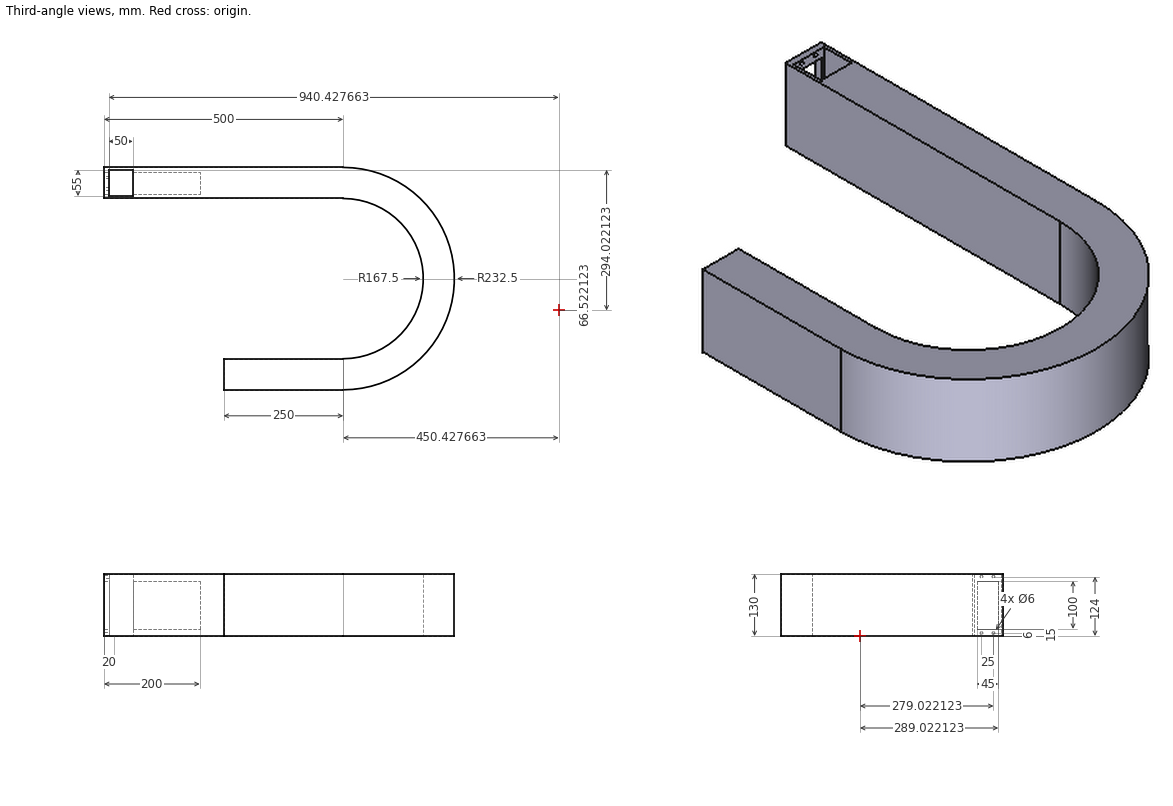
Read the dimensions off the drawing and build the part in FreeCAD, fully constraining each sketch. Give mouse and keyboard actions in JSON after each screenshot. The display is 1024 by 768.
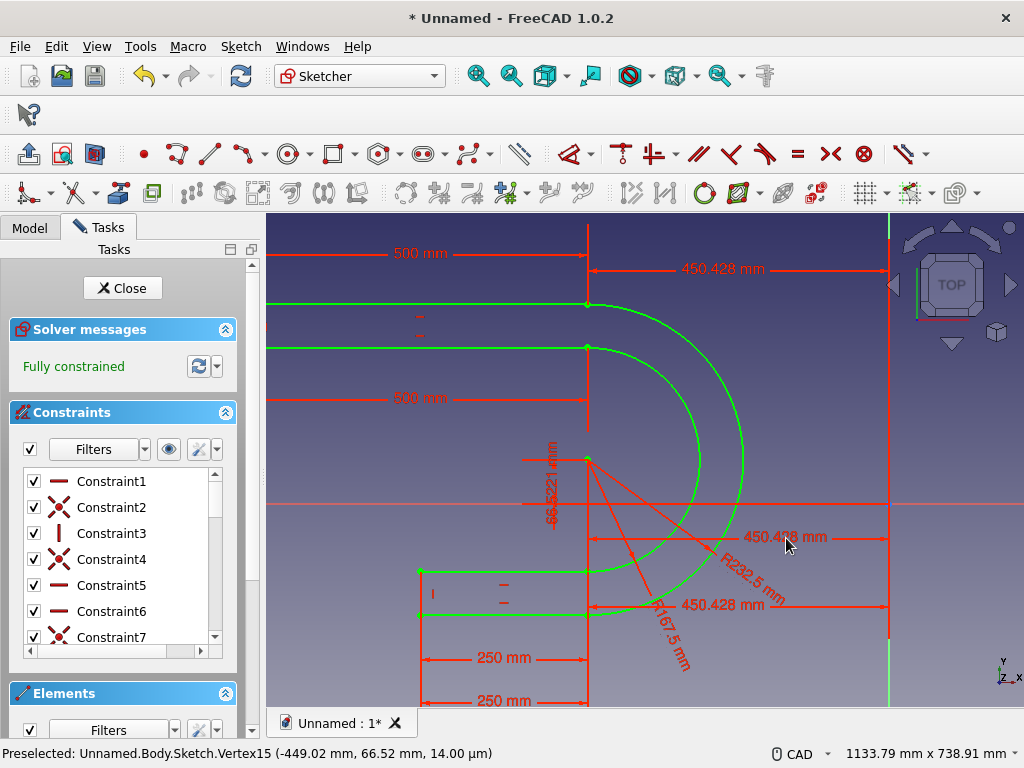
{"action": "left_click", "coordinate": [123, 288]}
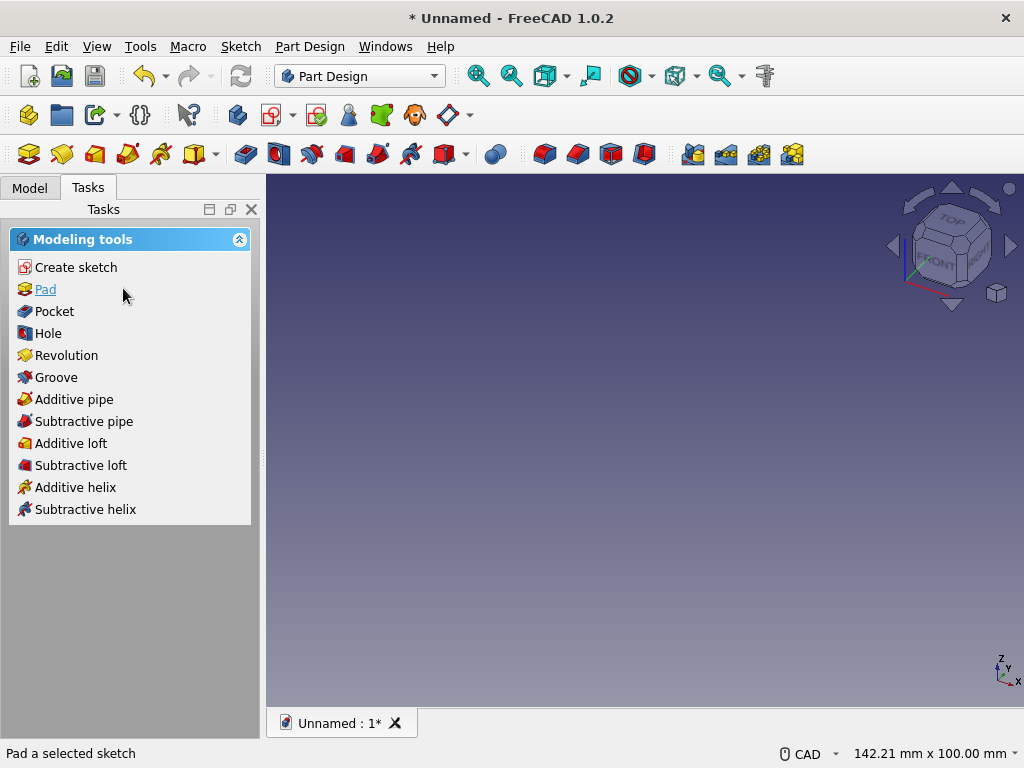
{"action": "left_click", "coordinate": [29, 154]}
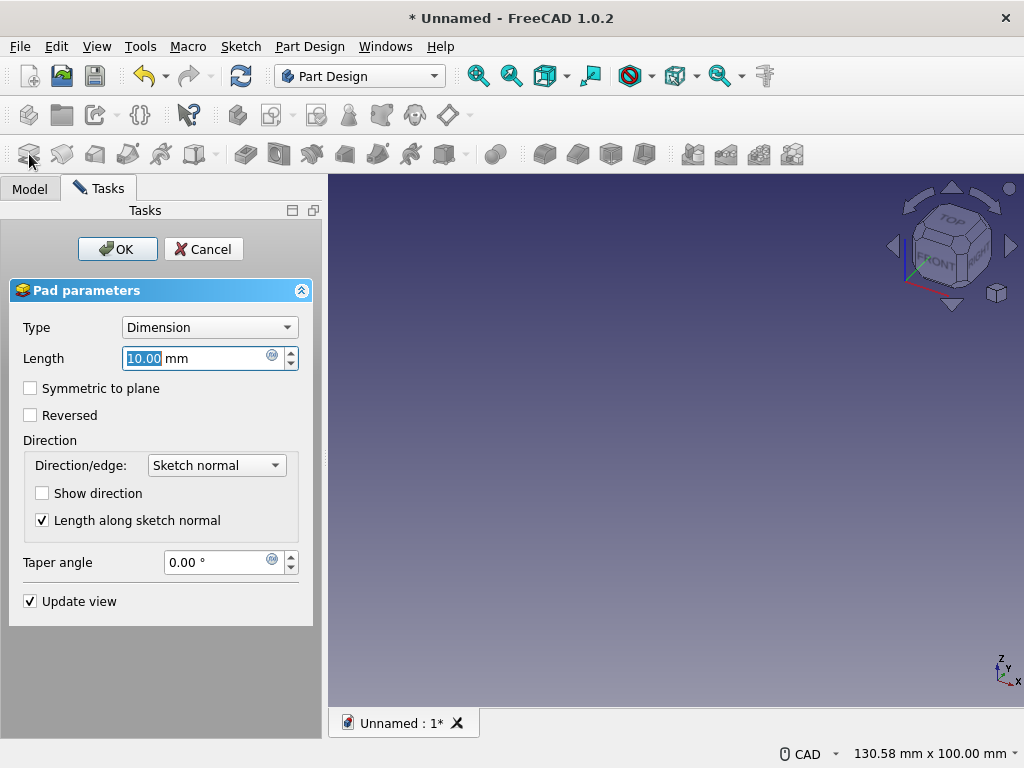
{"action": "type", "text": "130"}
{"action": "key", "text": "Tab"}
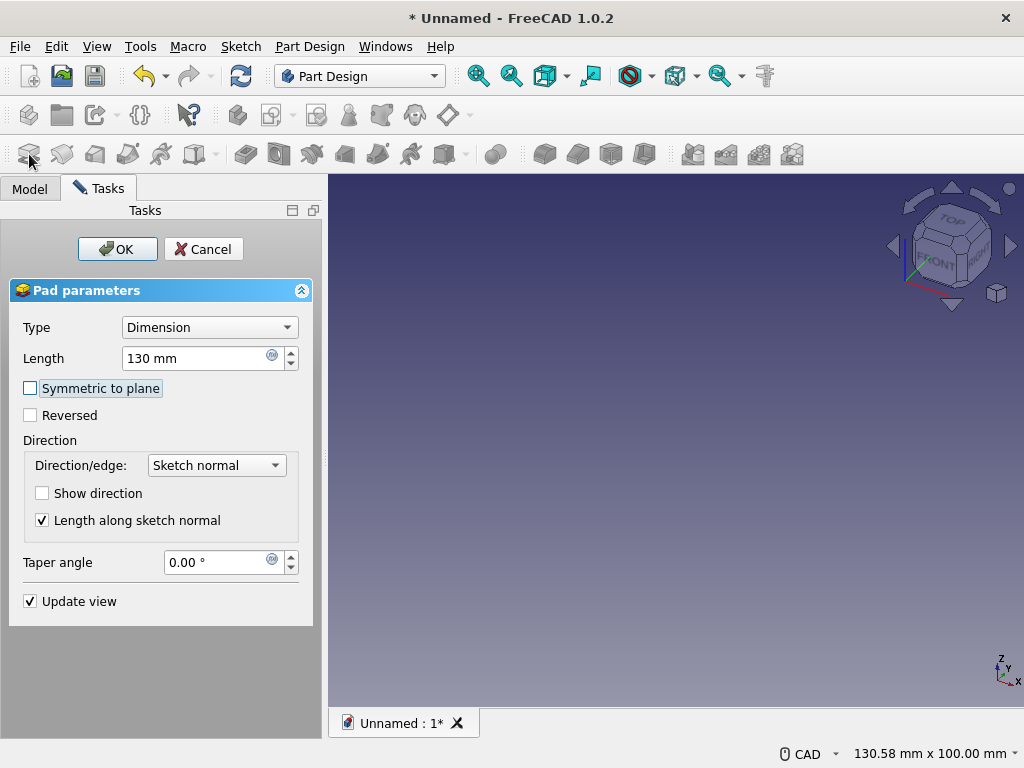
{"action": "left_click", "coordinate": [118, 249]}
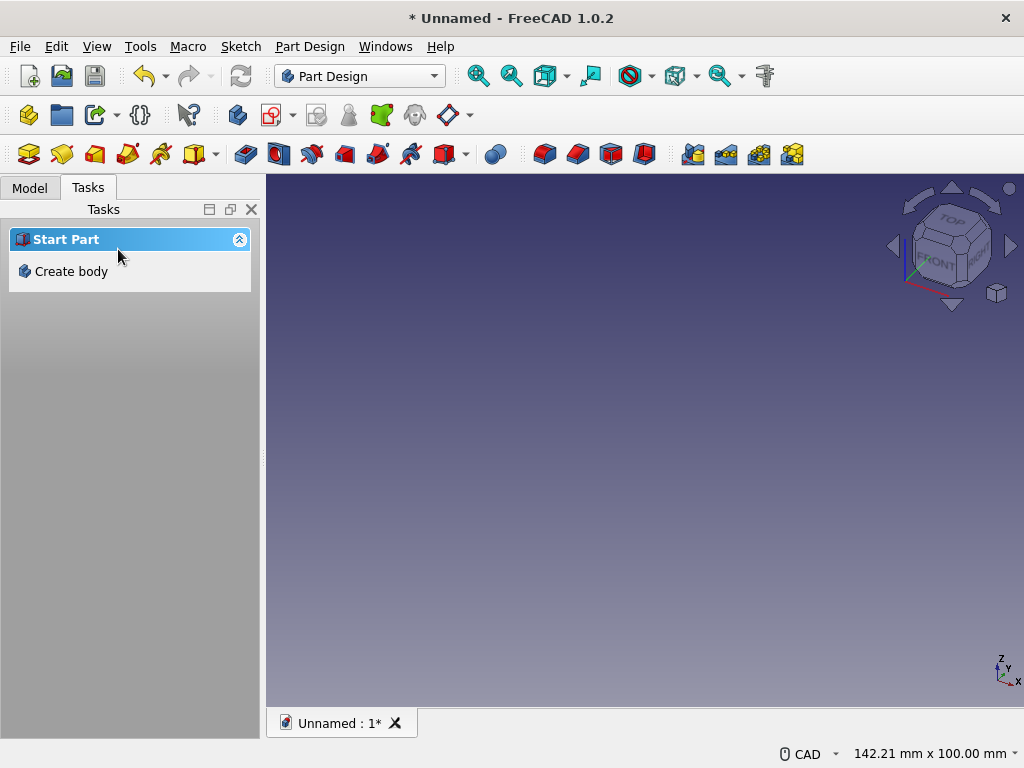
{"action": "key", "text": "v f"}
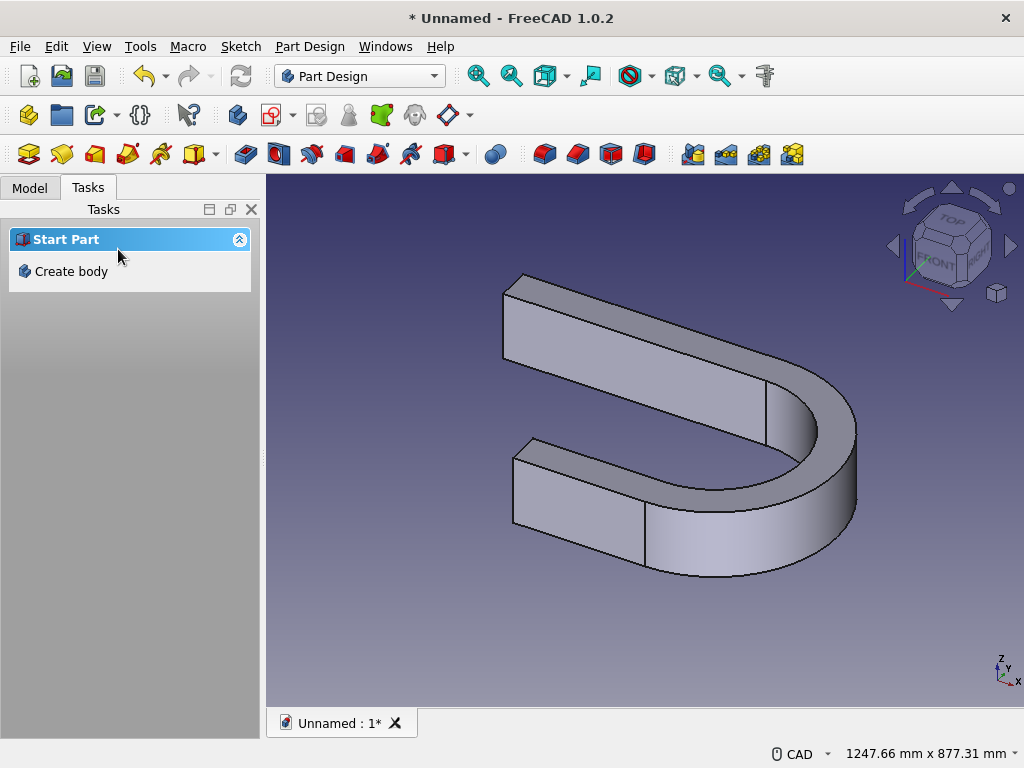
{"action": "key", "text": "6"}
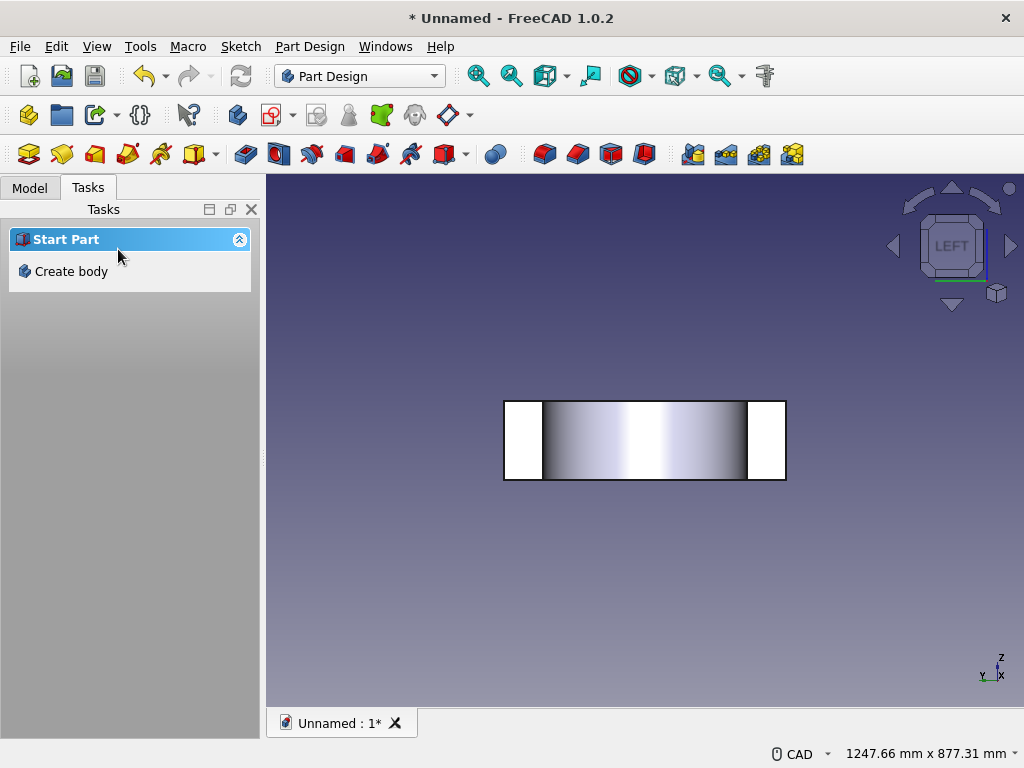
{"action": "left_click", "coordinate": [479, 76]}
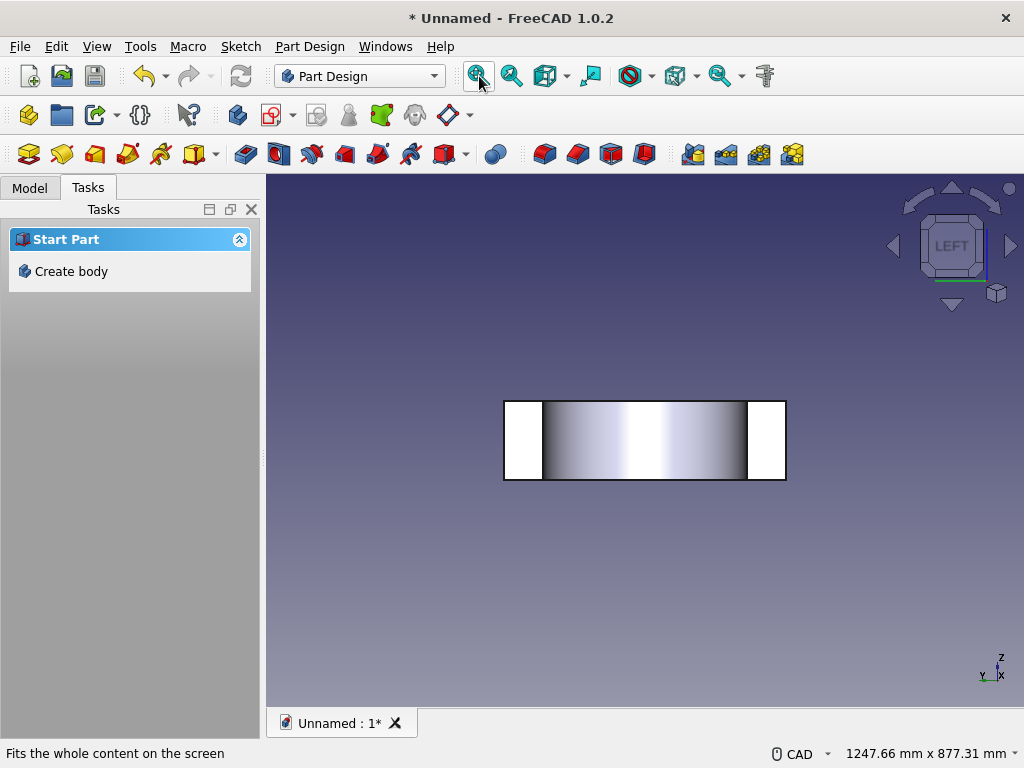
{"action": "left_click", "coordinate": [523, 428]}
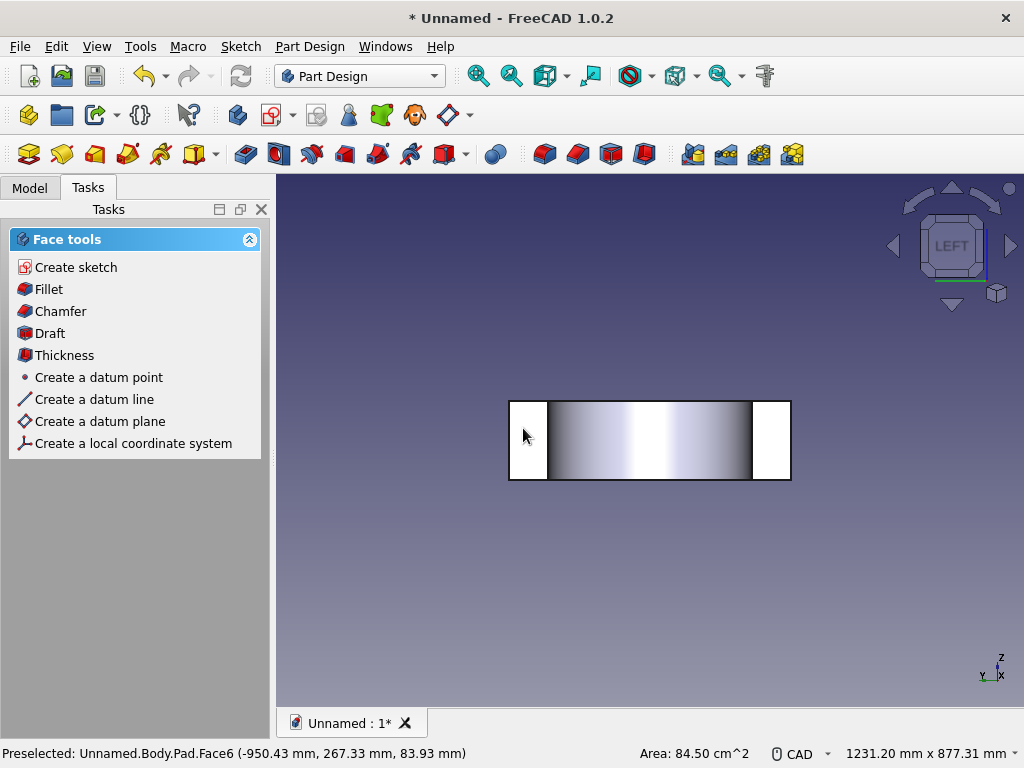
{"action": "left_click", "coordinate": [270, 116]}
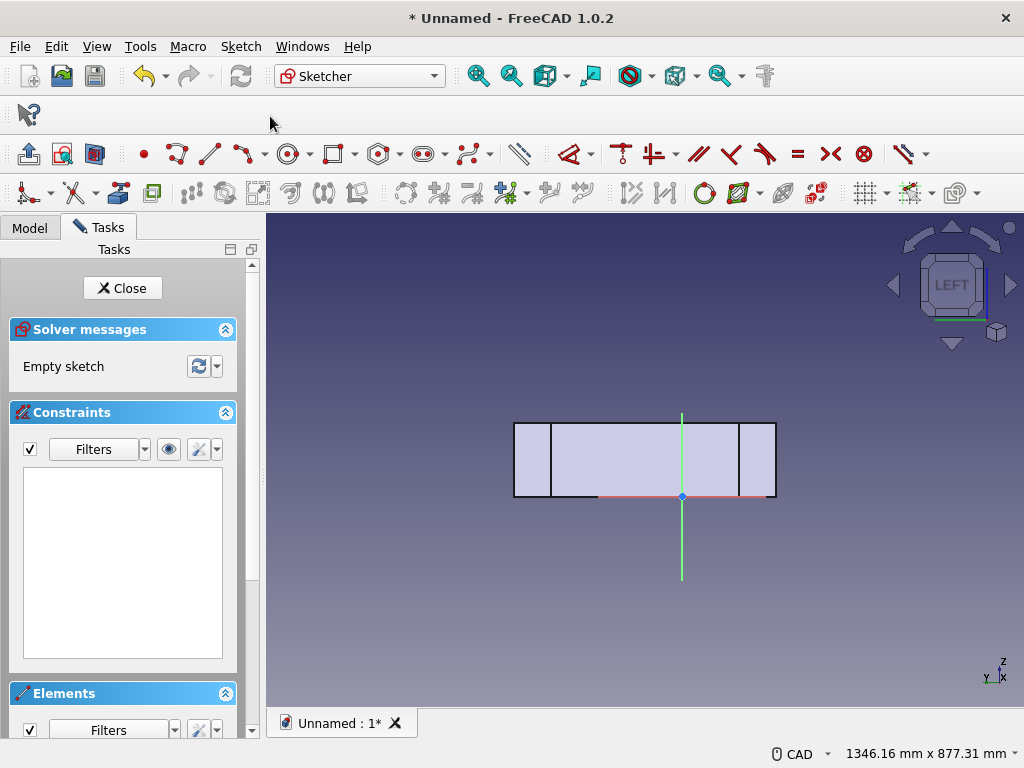
{"action": "scroll", "coordinate": [619, 461], "scroll_direction": "up", "scroll_amount": 5}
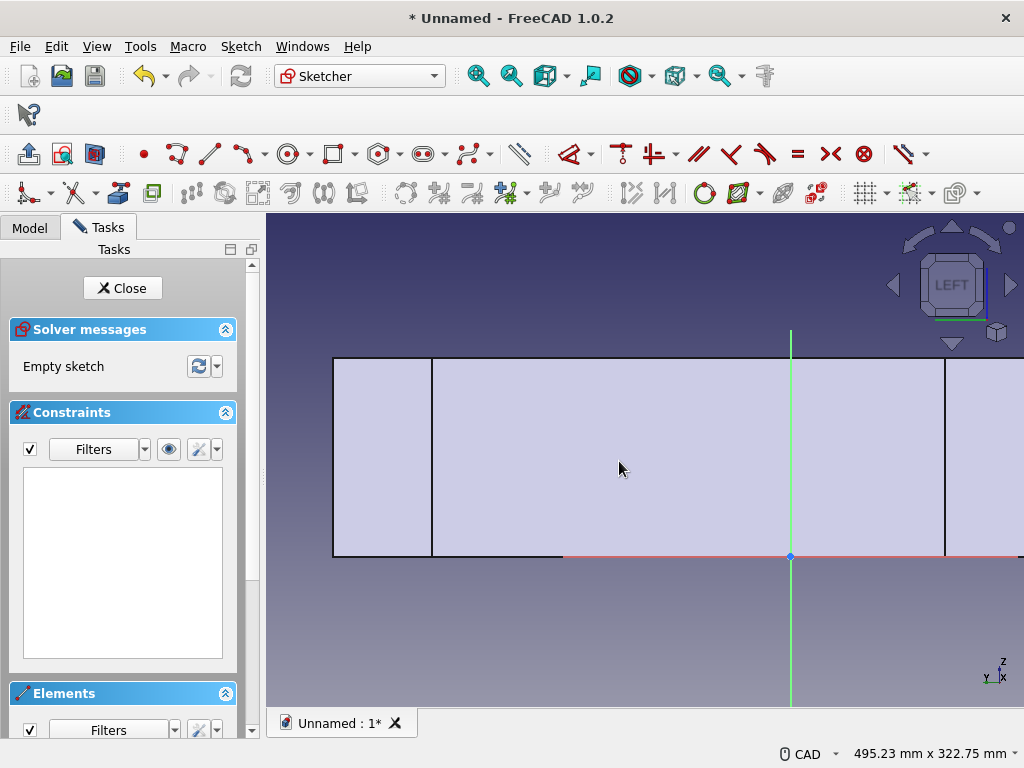
{"action": "key", "text": "g c"}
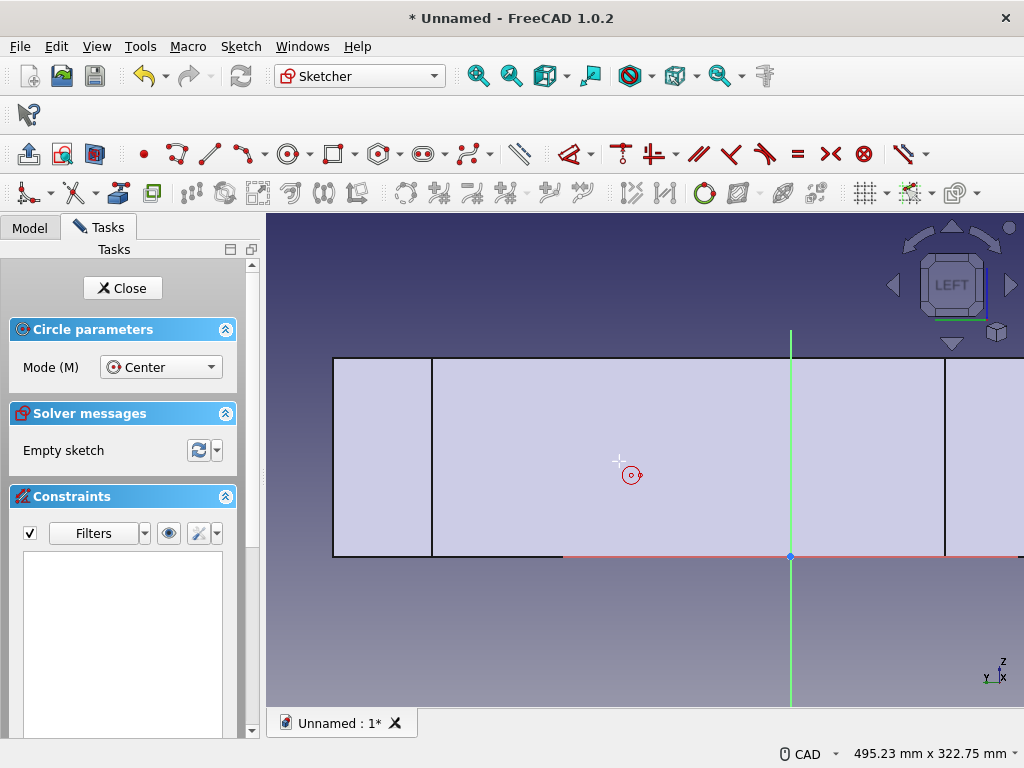
{"action": "scroll", "coordinate": [364, 548], "scroll_direction": "up", "scroll_amount": 8}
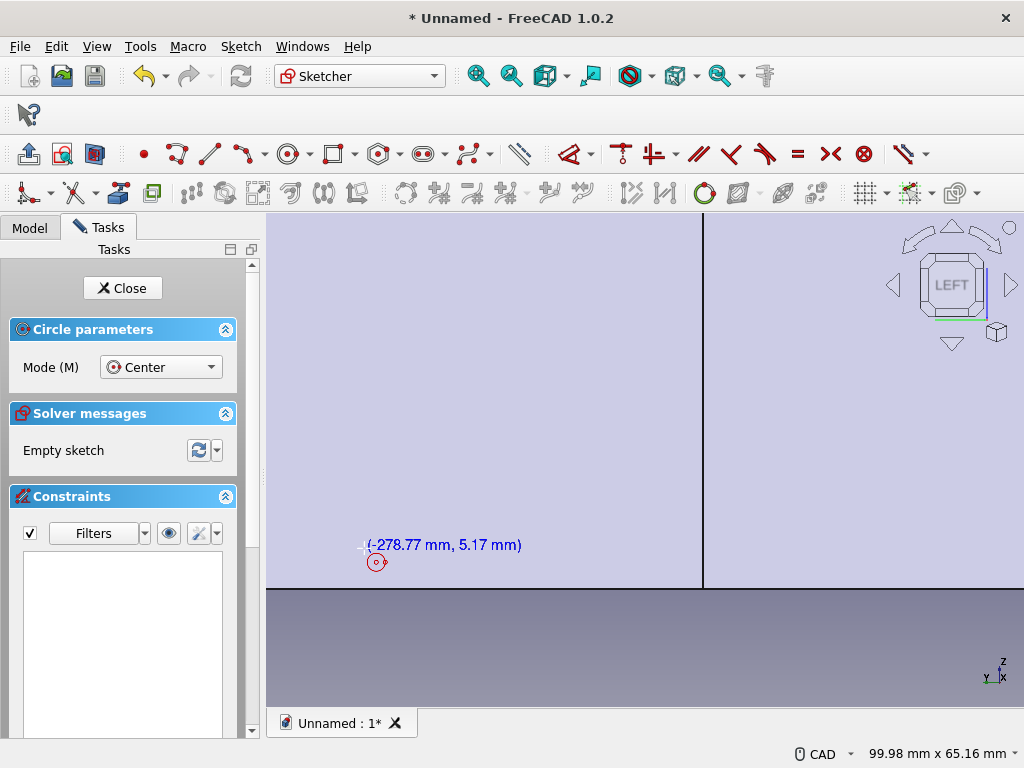
{"action": "left_click", "coordinate": [362, 544]}